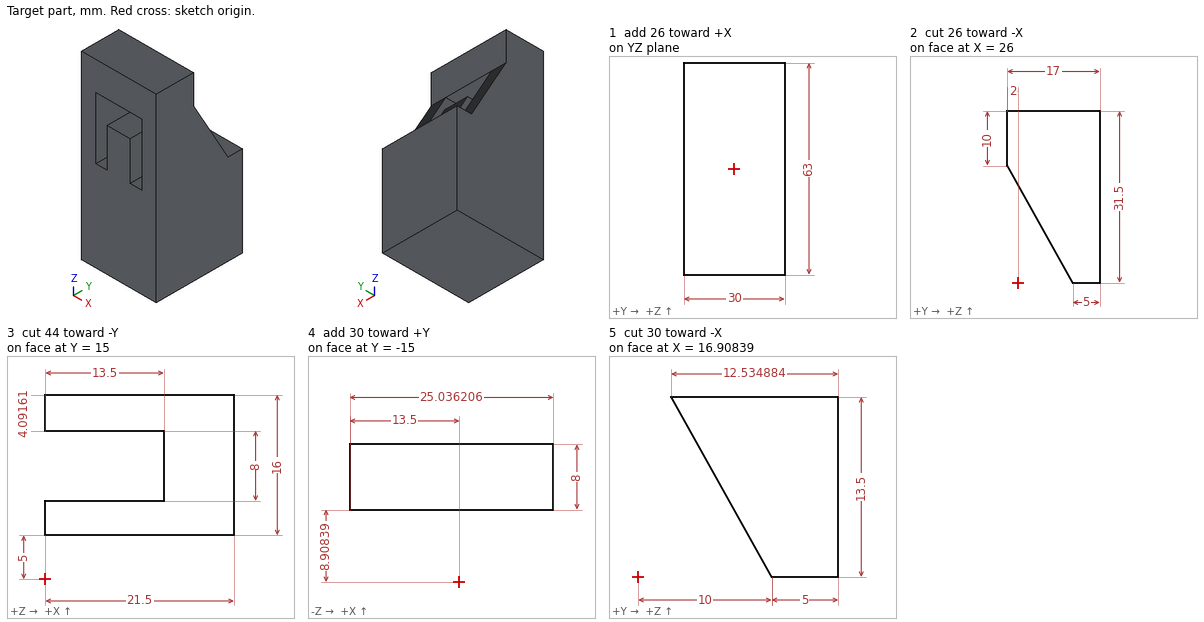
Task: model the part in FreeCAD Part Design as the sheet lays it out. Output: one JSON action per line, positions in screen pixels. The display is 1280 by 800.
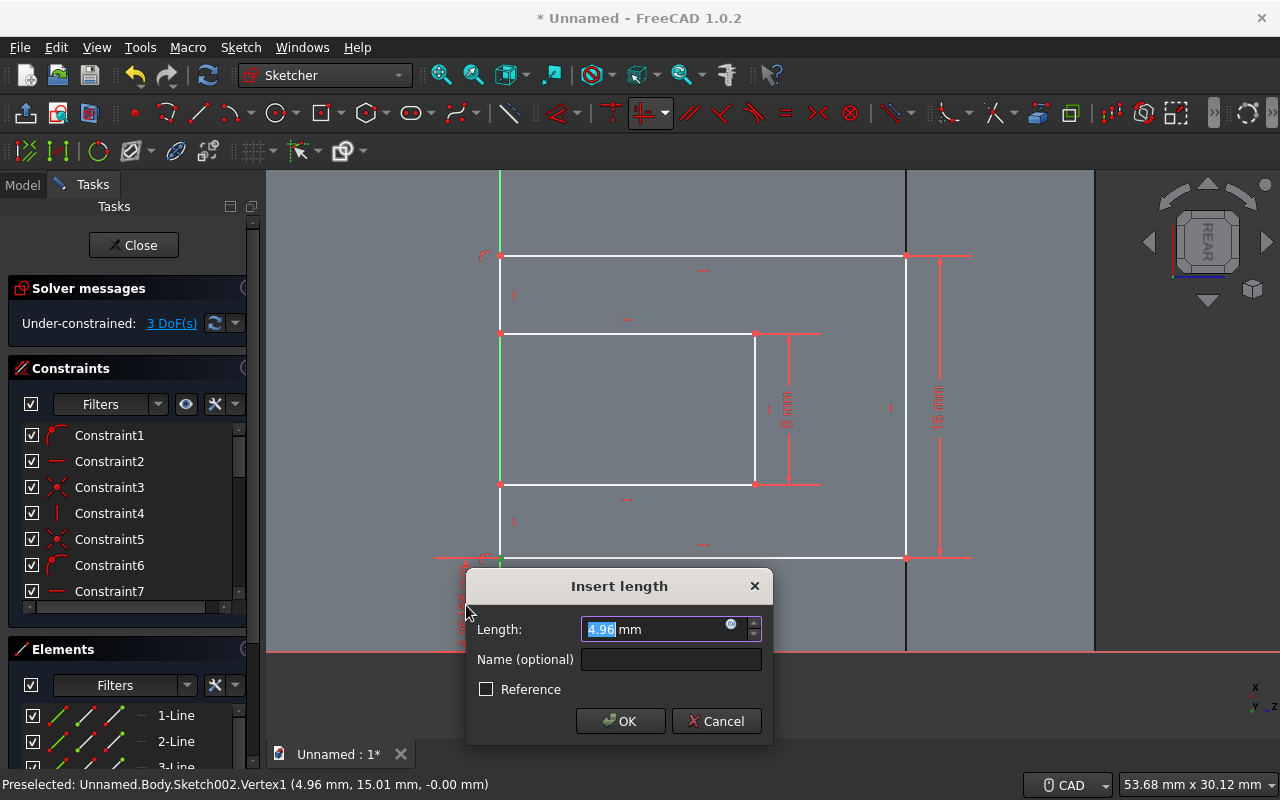
{"action": "type", "text": "5"}
{"action": "key", "text": "Return"}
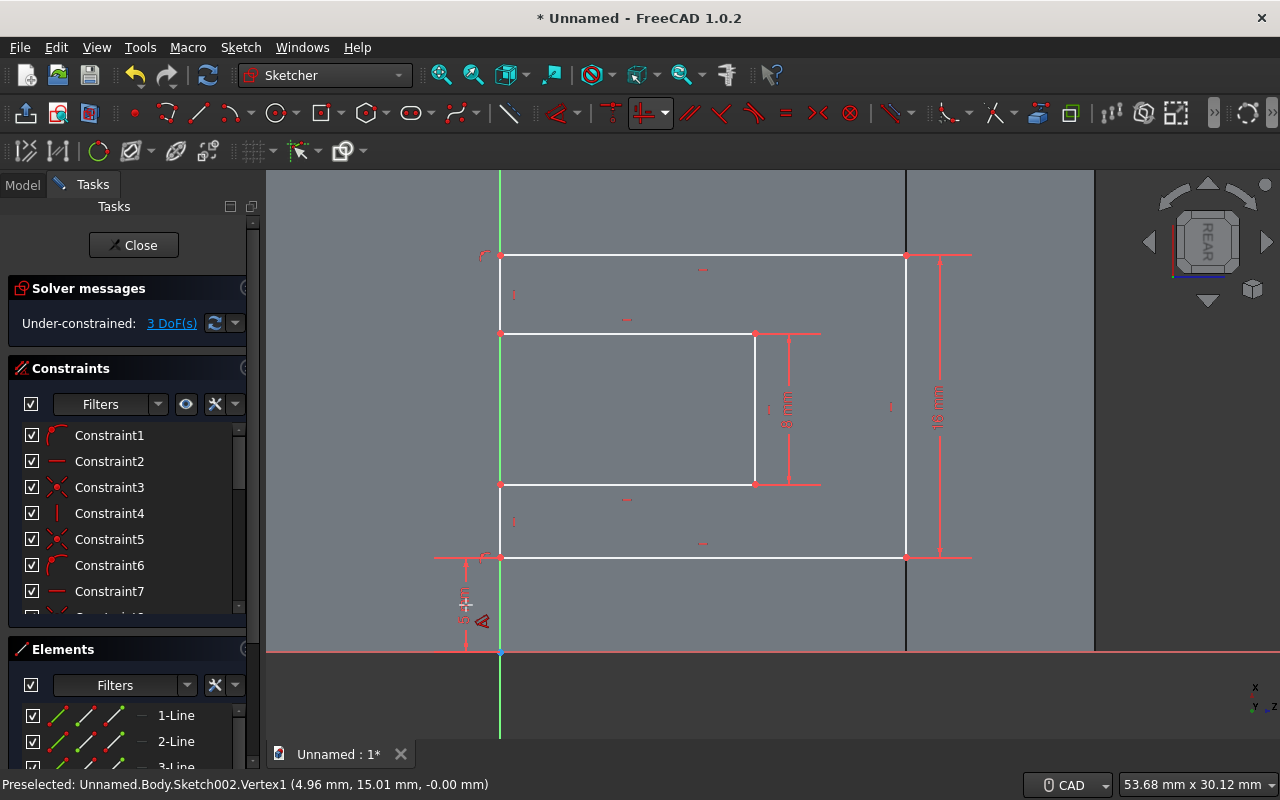
{"action": "left_click", "coordinate": [622, 558]}
{"action": "left_click", "coordinate": [703, 592]}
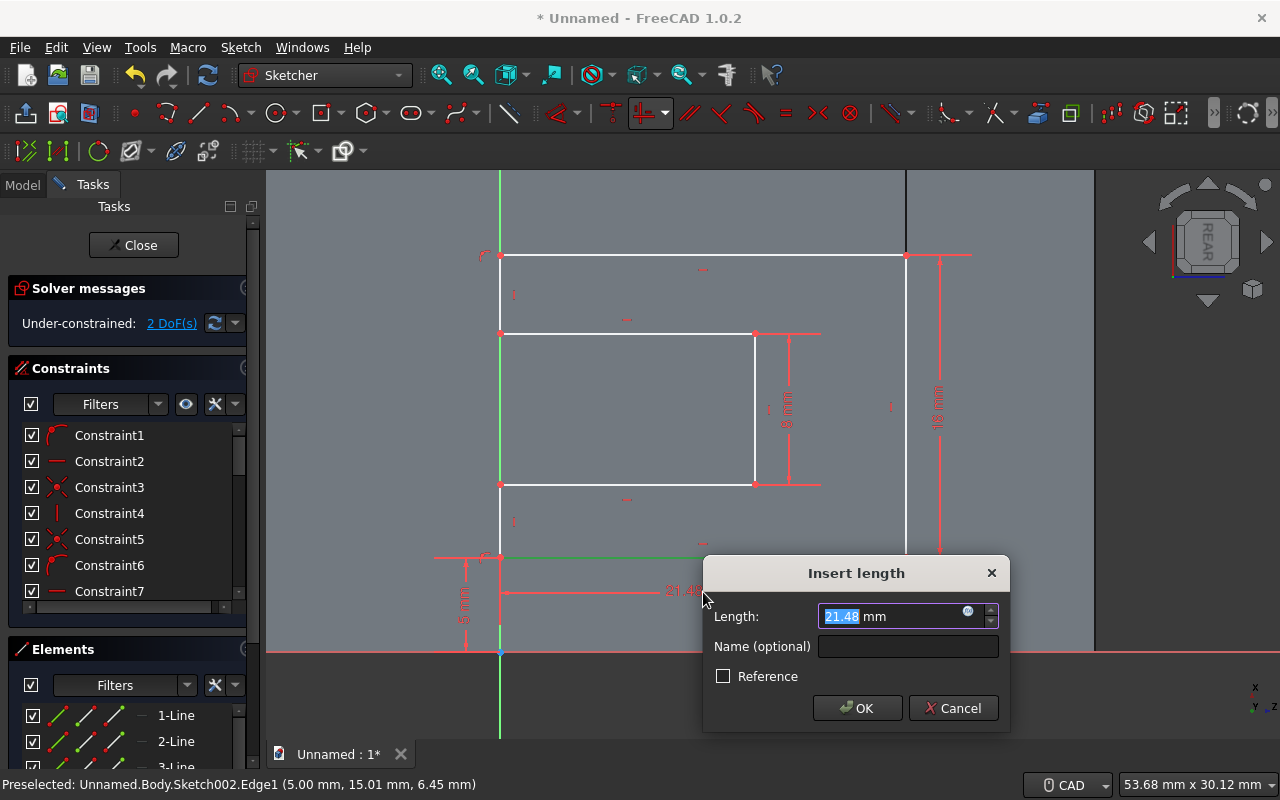
{"action": "type", "text": "21.5"}
{"action": "key", "text": "Return"}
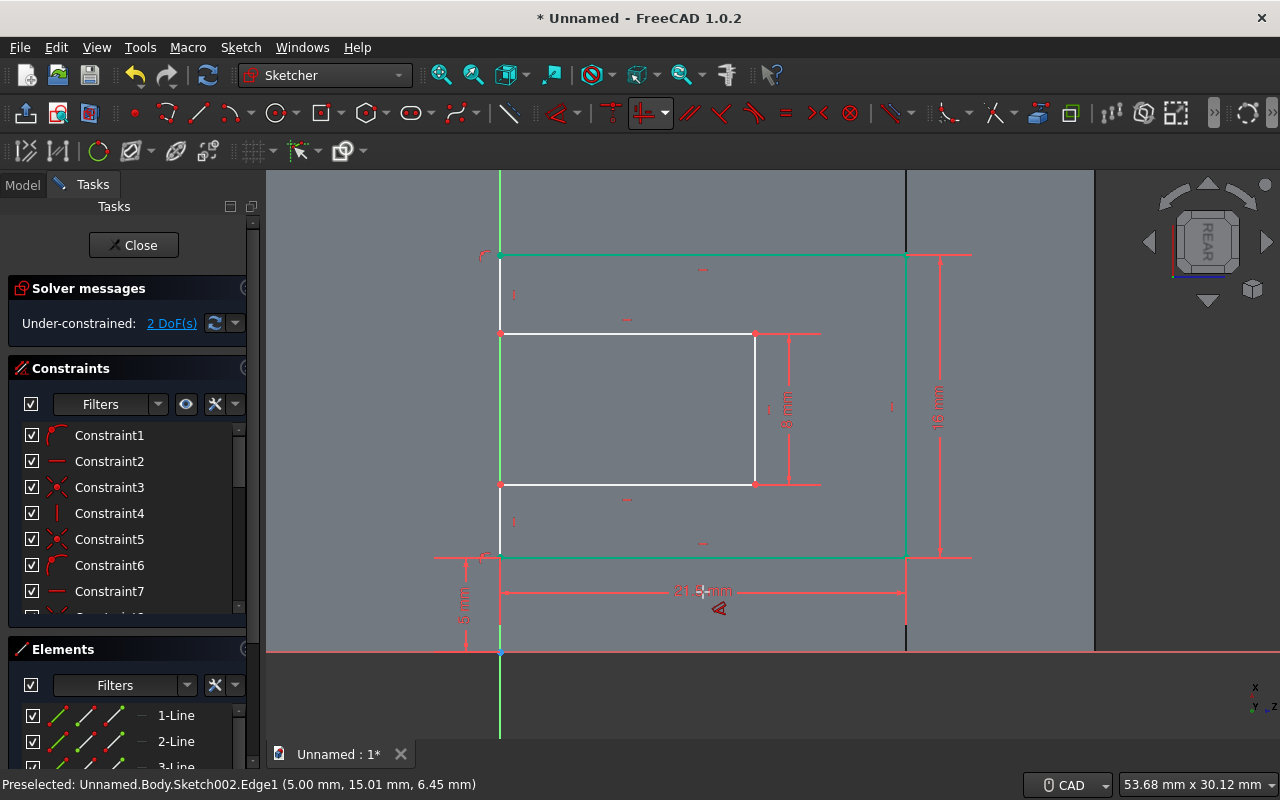
{"action": "left_click", "coordinate": [577, 334]}
{"action": "left_click", "coordinate": [628, 300]}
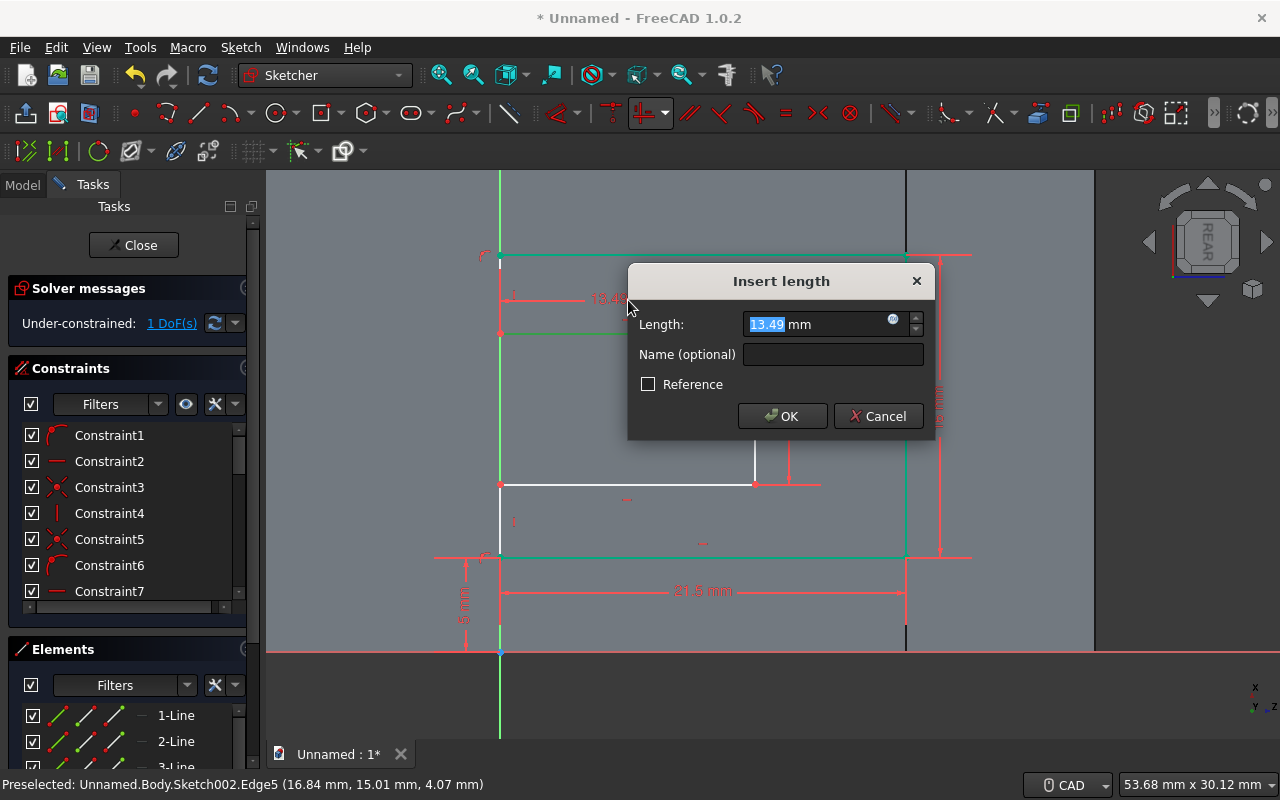
{"action": "type", "text": "13.5"}
{"action": "key", "text": "Return"}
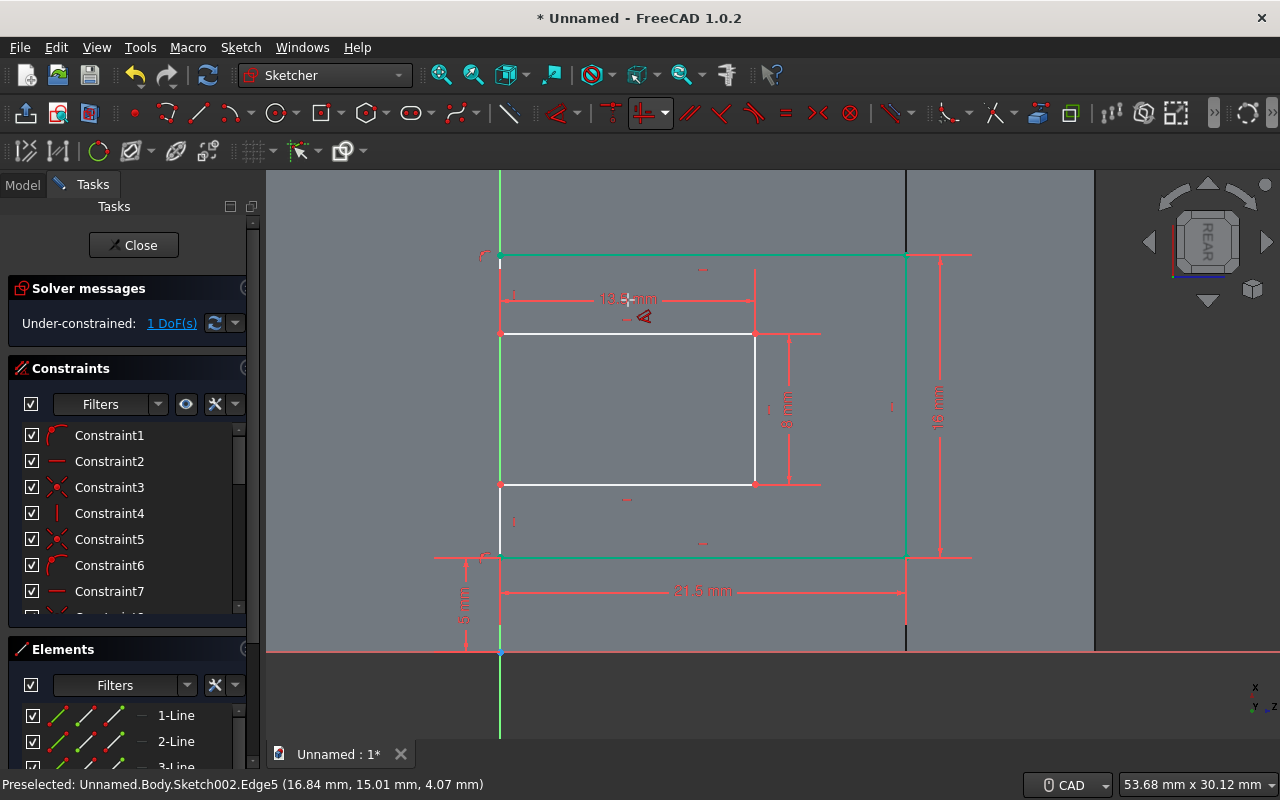
{"action": "left_click", "coordinate": [500, 279]}
{"action": "left_click", "coordinate": [466, 295]}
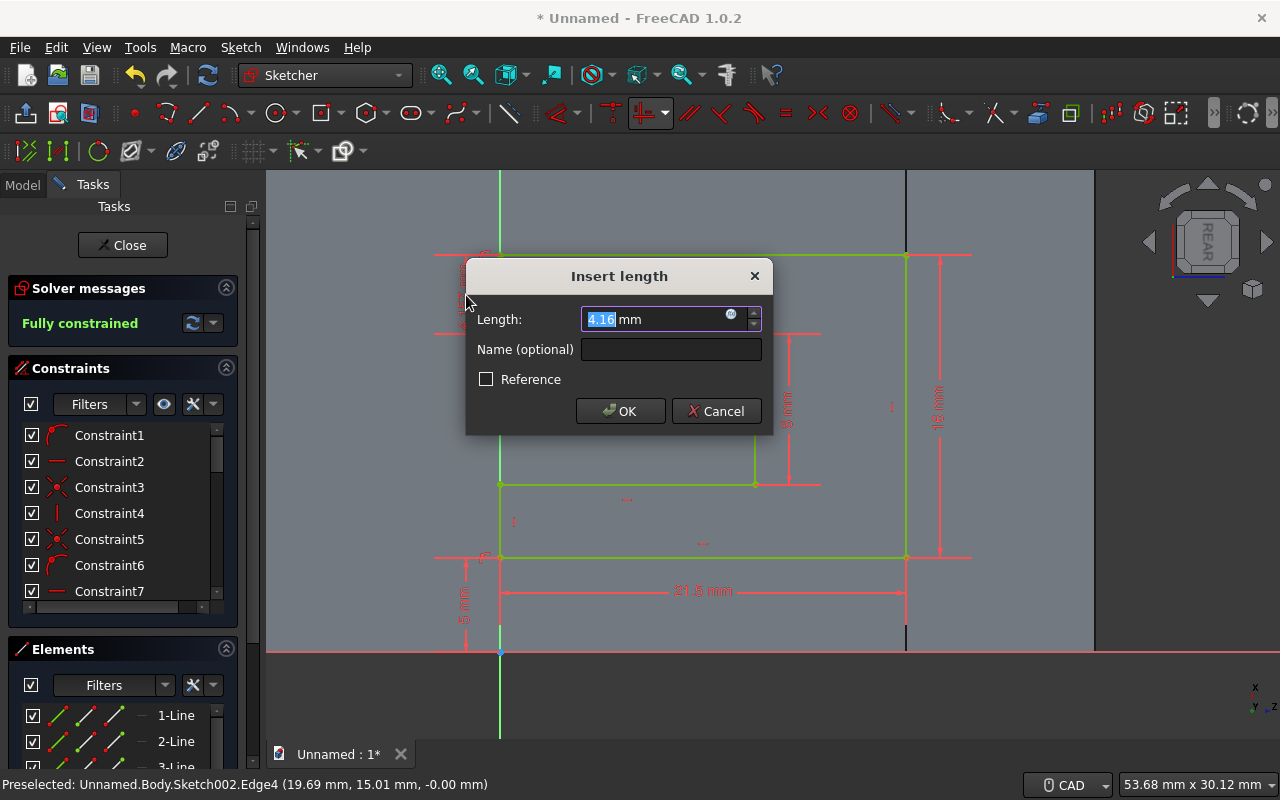
{"action": "type", "text": "4.09161"}
{"action": "key", "text": "Return"}
{"action": "key", "text": "Escape"}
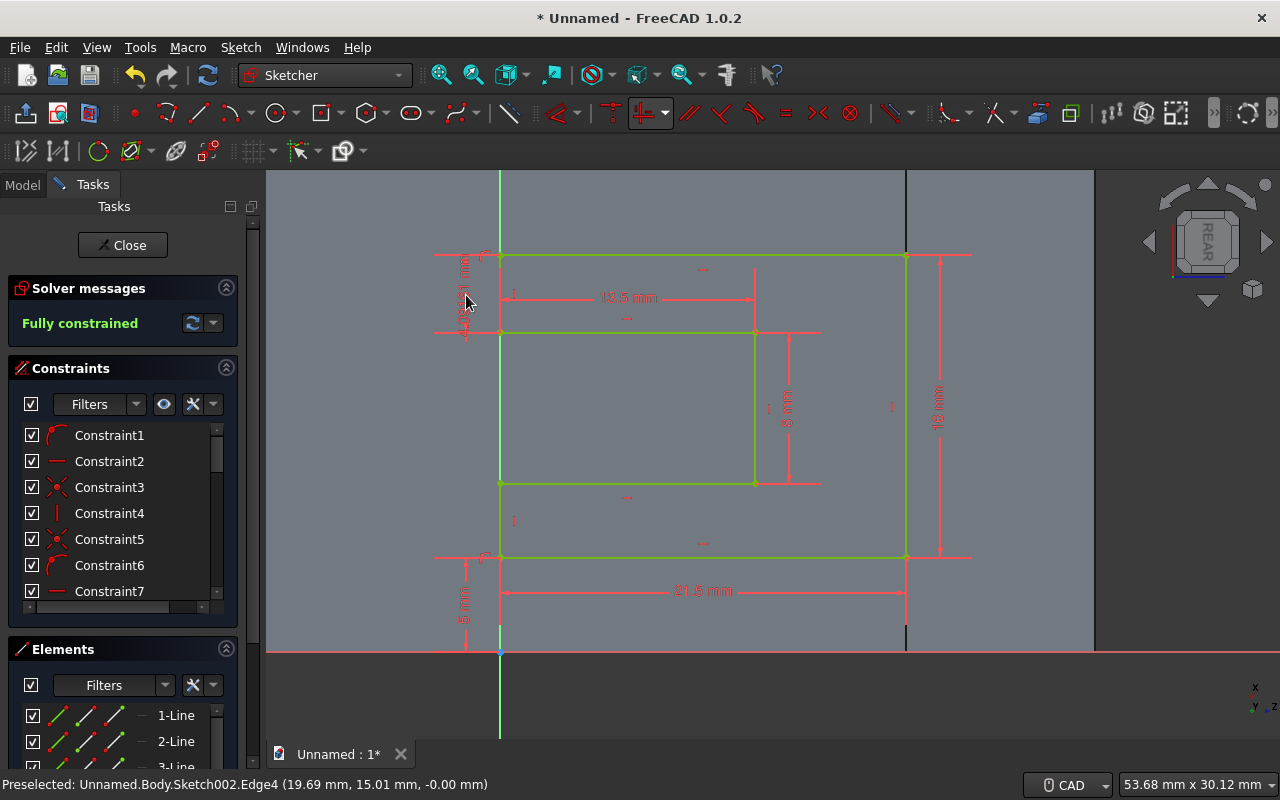
{"action": "left_click", "coordinate": [123, 245]}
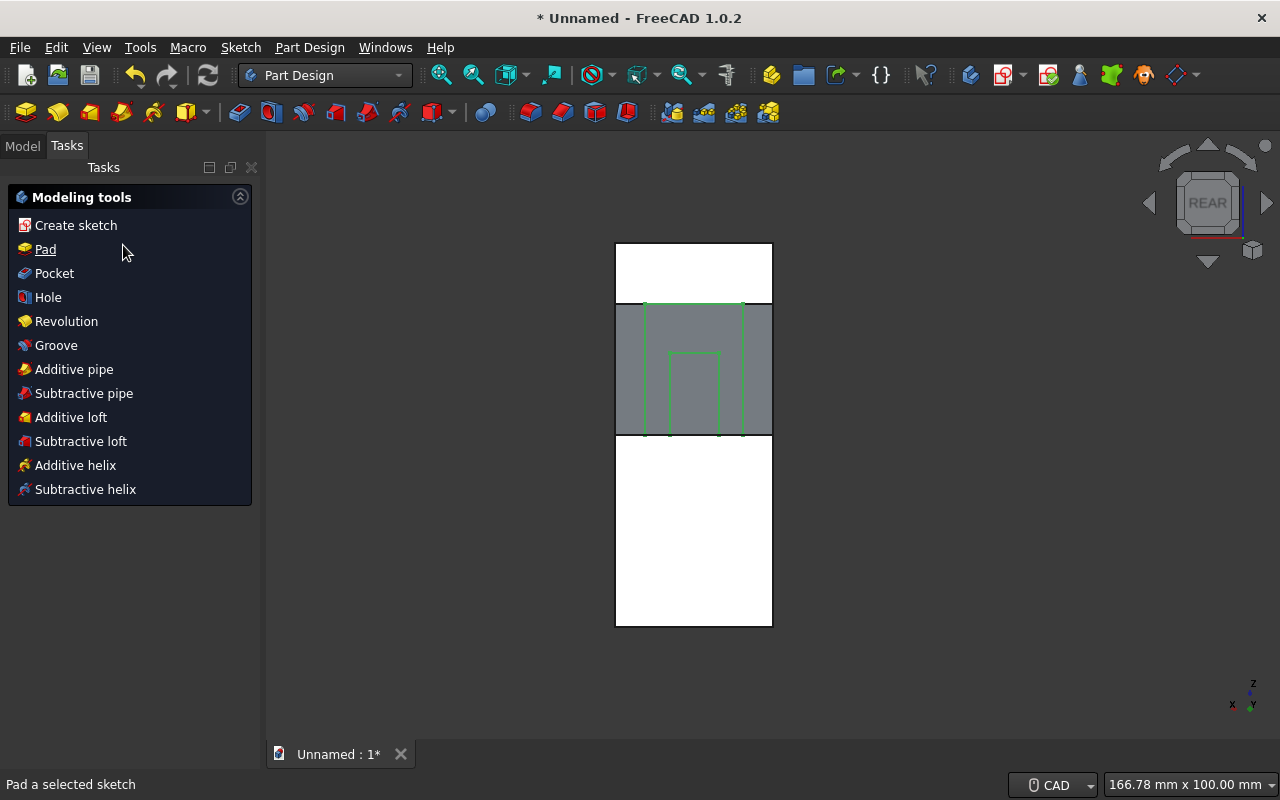
{"action": "left_click", "coordinate": [240, 112]}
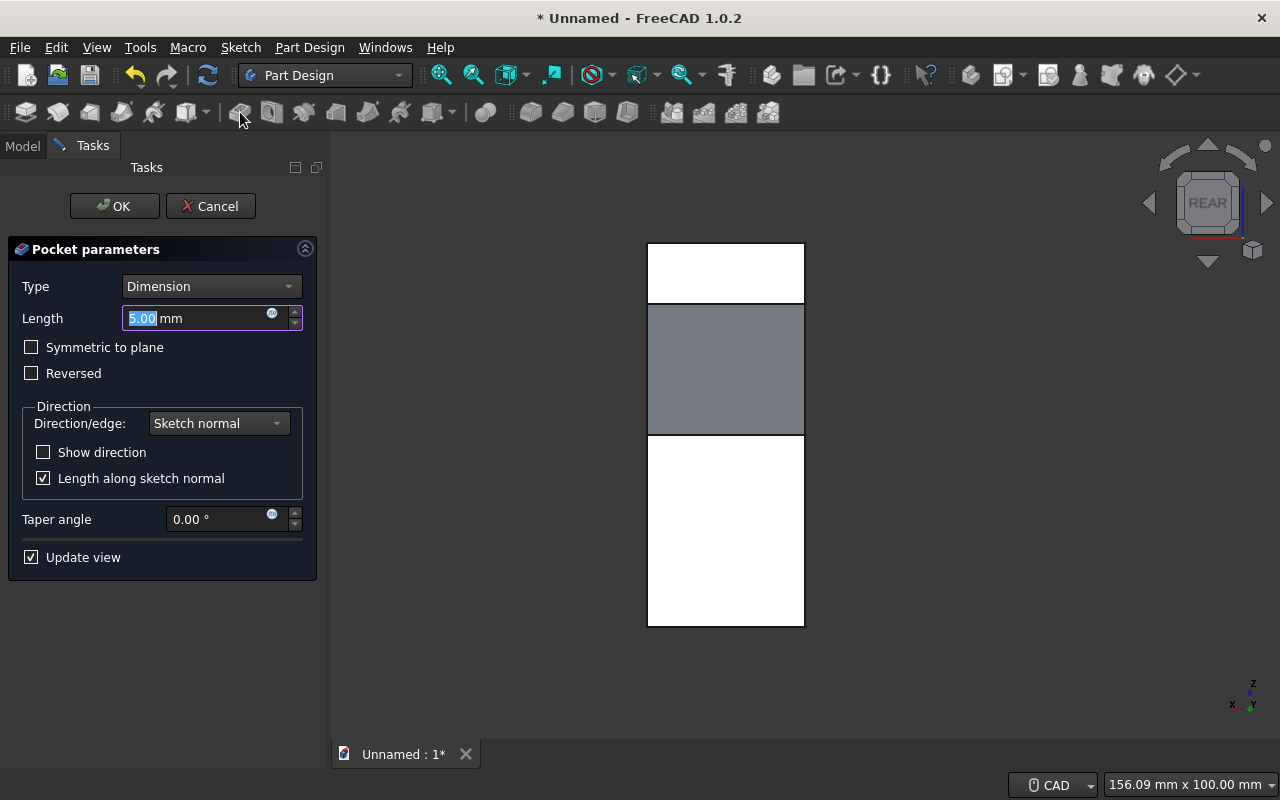
{"action": "type", "text": "44"}
{"action": "key", "text": "Tab"}